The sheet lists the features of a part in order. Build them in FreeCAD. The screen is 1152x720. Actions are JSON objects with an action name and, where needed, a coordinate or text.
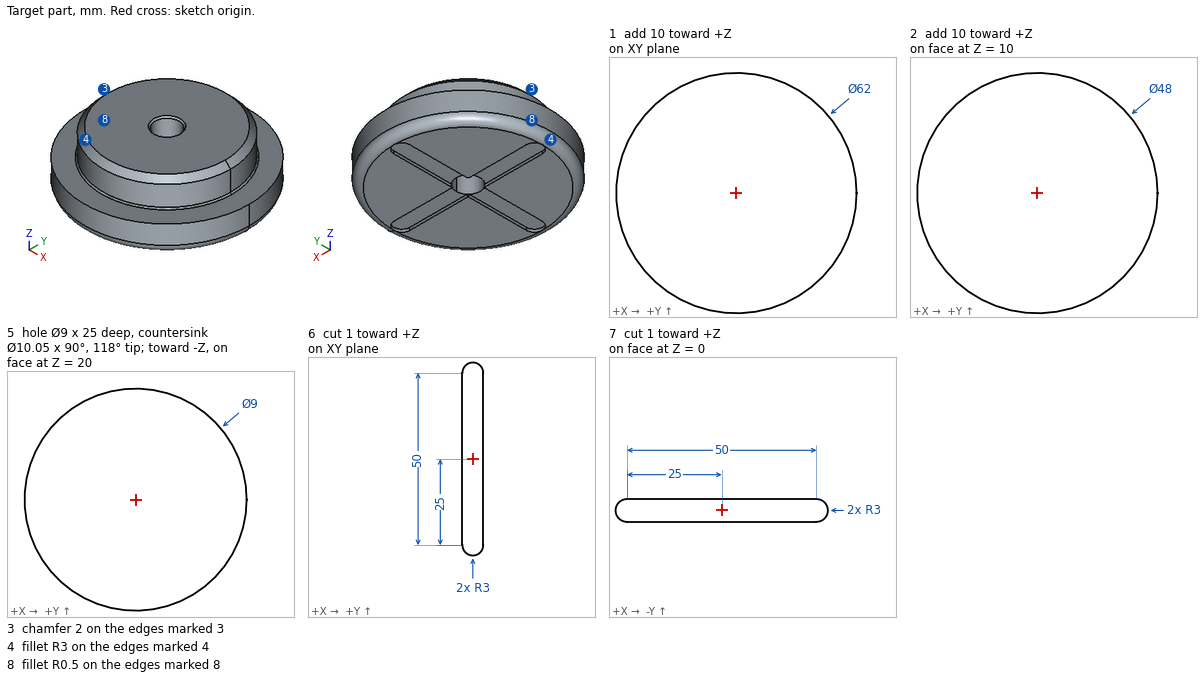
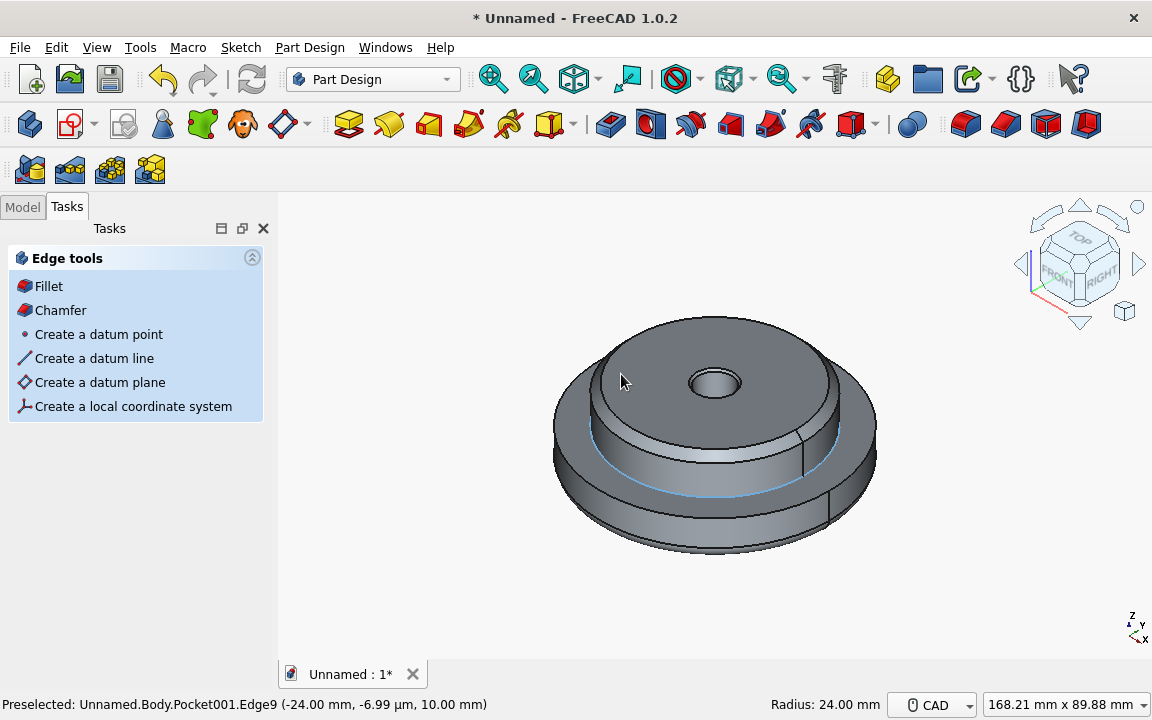
{"action": "left_click", "coordinate": [966, 124]}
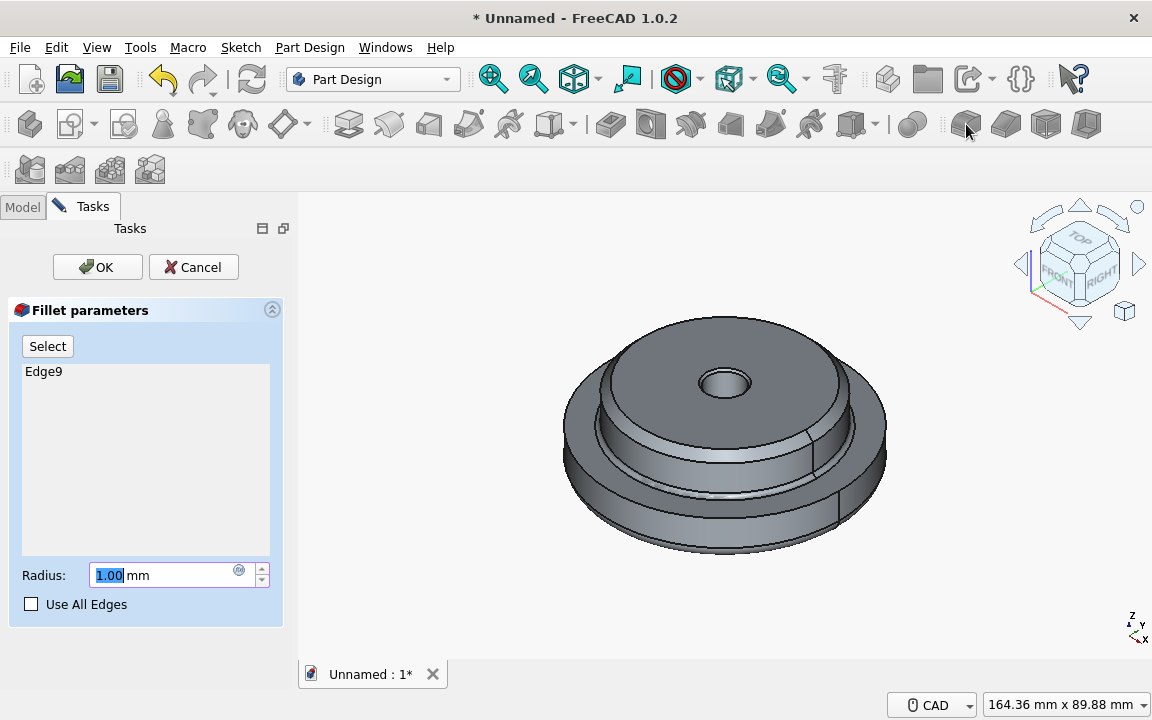
{"action": "type", "text": "0.5"}
{"action": "key", "text": "Tab"}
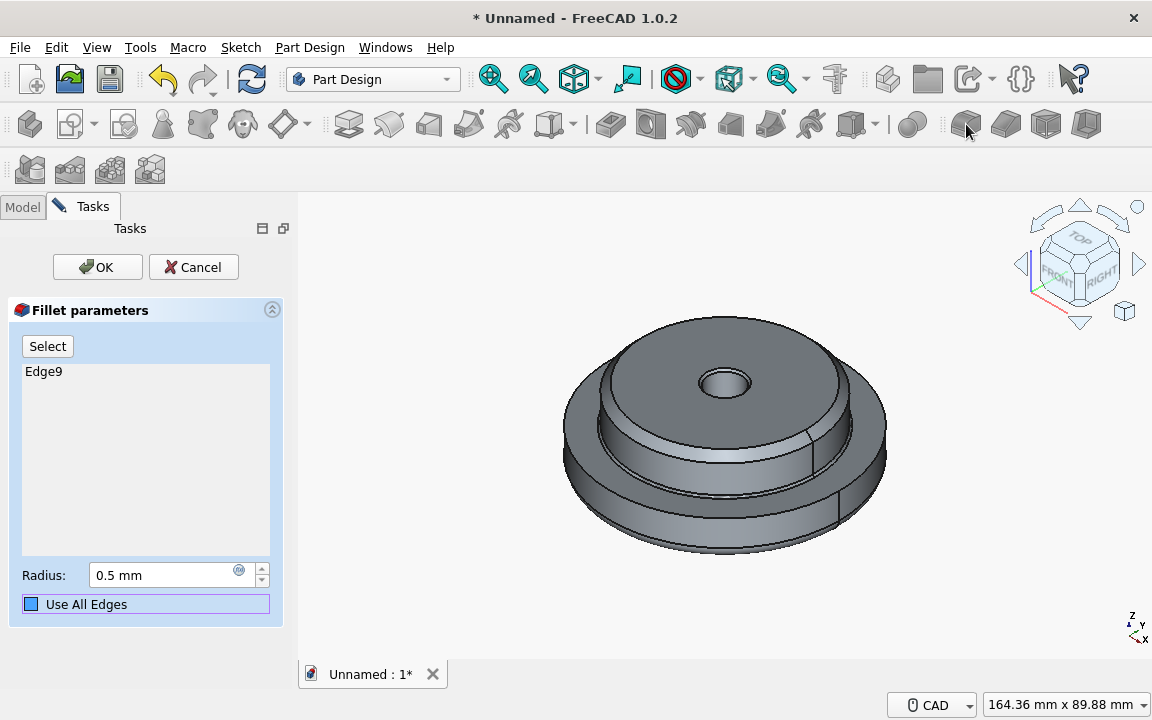
{"action": "left_click", "coordinate": [98, 267]}